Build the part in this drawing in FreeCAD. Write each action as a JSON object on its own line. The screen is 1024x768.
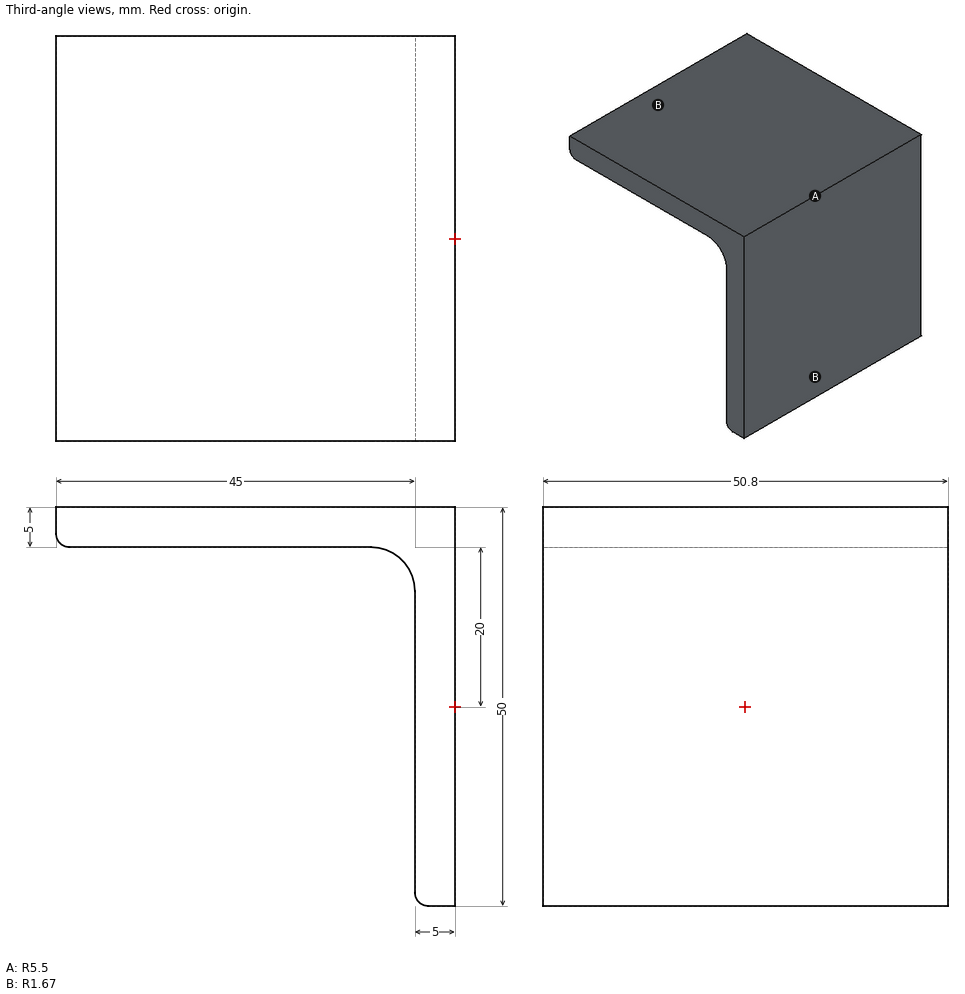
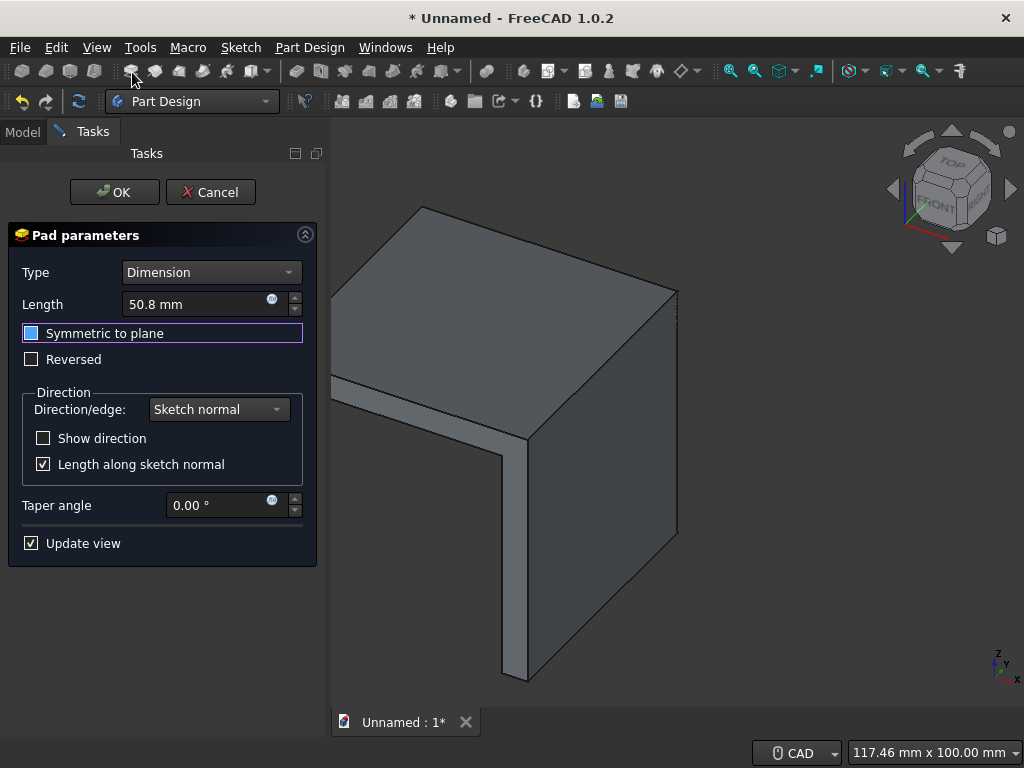
{"action": "left_click", "coordinate": [30, 333]}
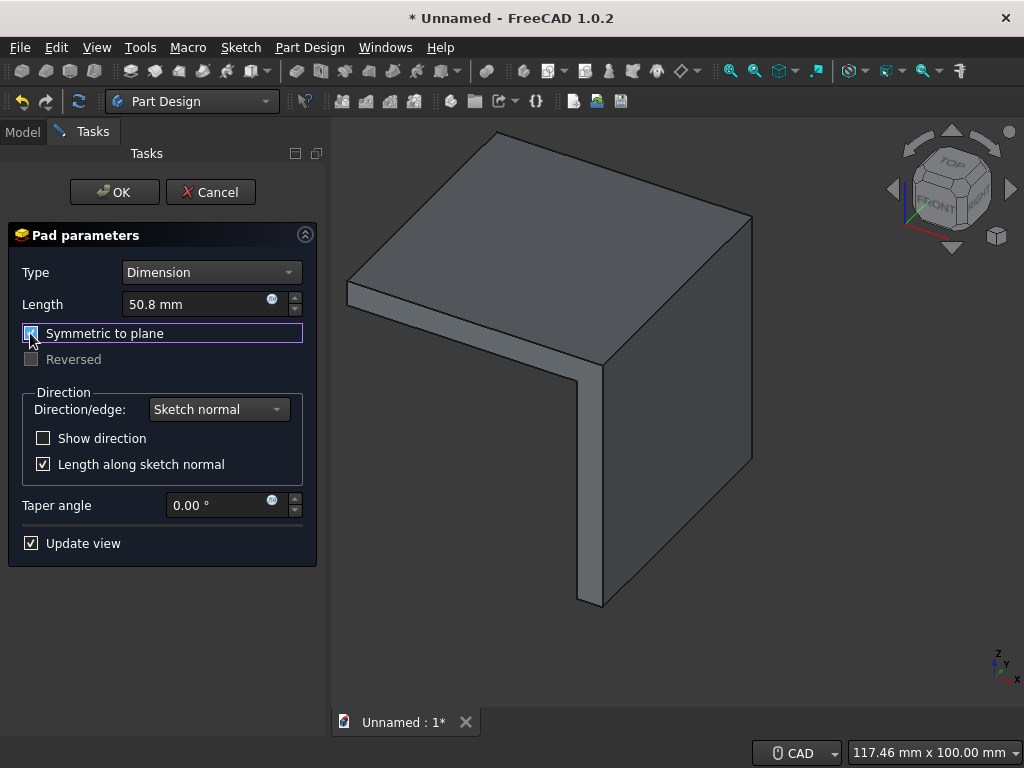
{"action": "left_click", "coordinate": [115, 192]}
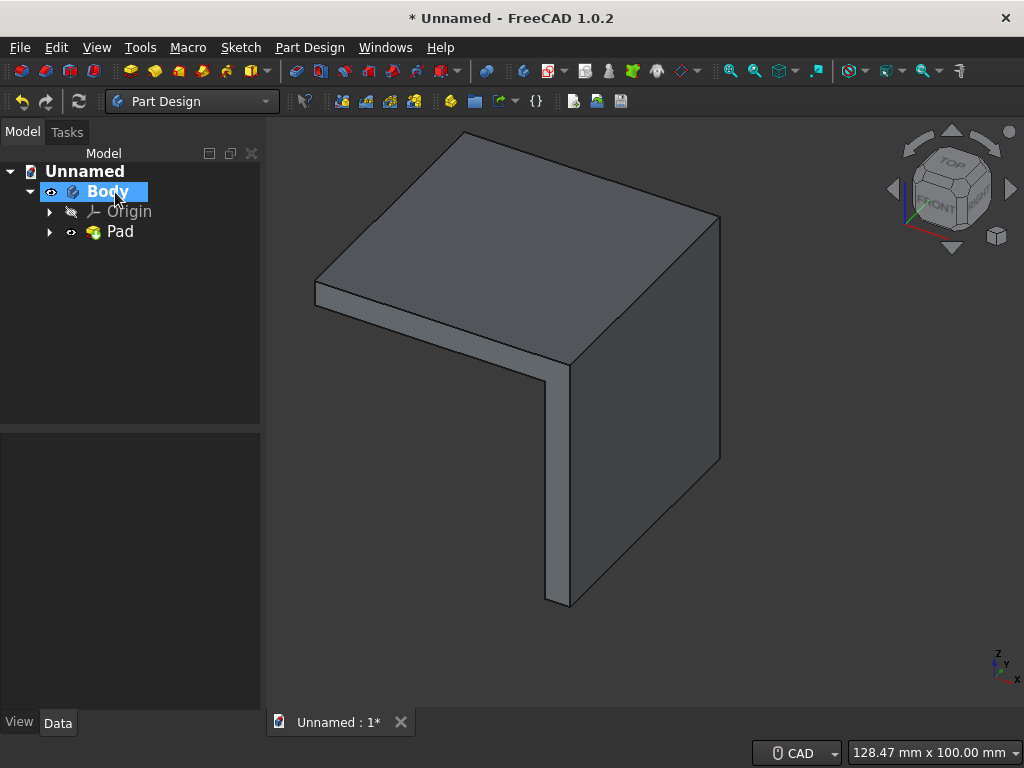
{"action": "key", "text": "0"}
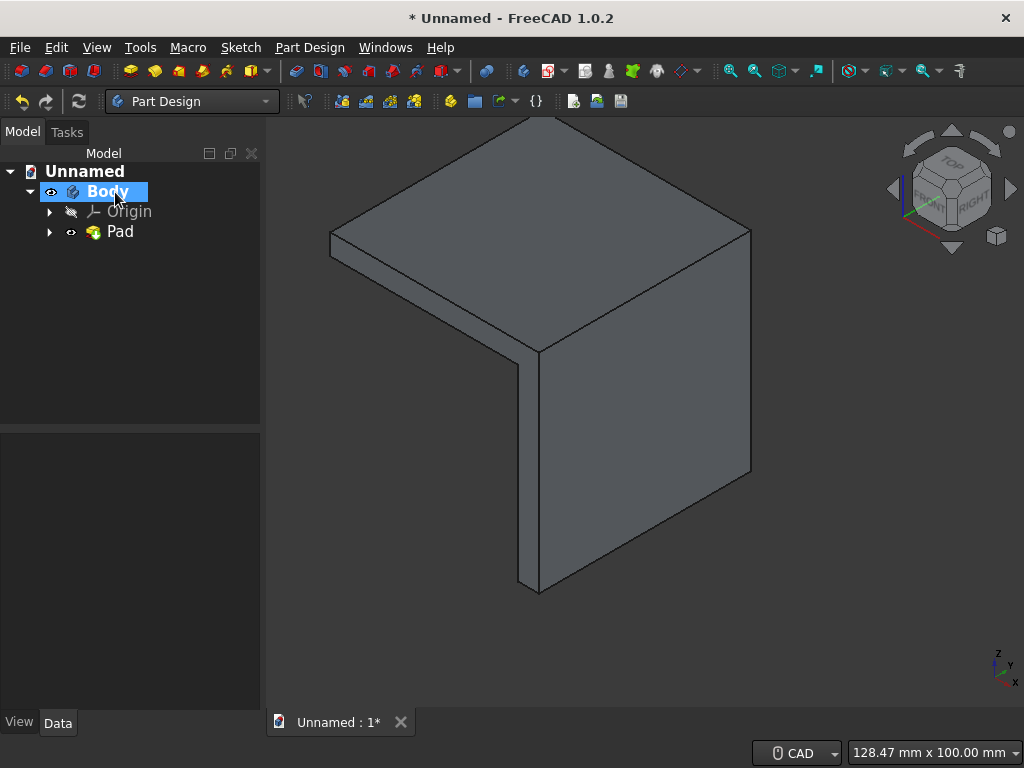
{"action": "left_click", "coordinate": [732, 72]}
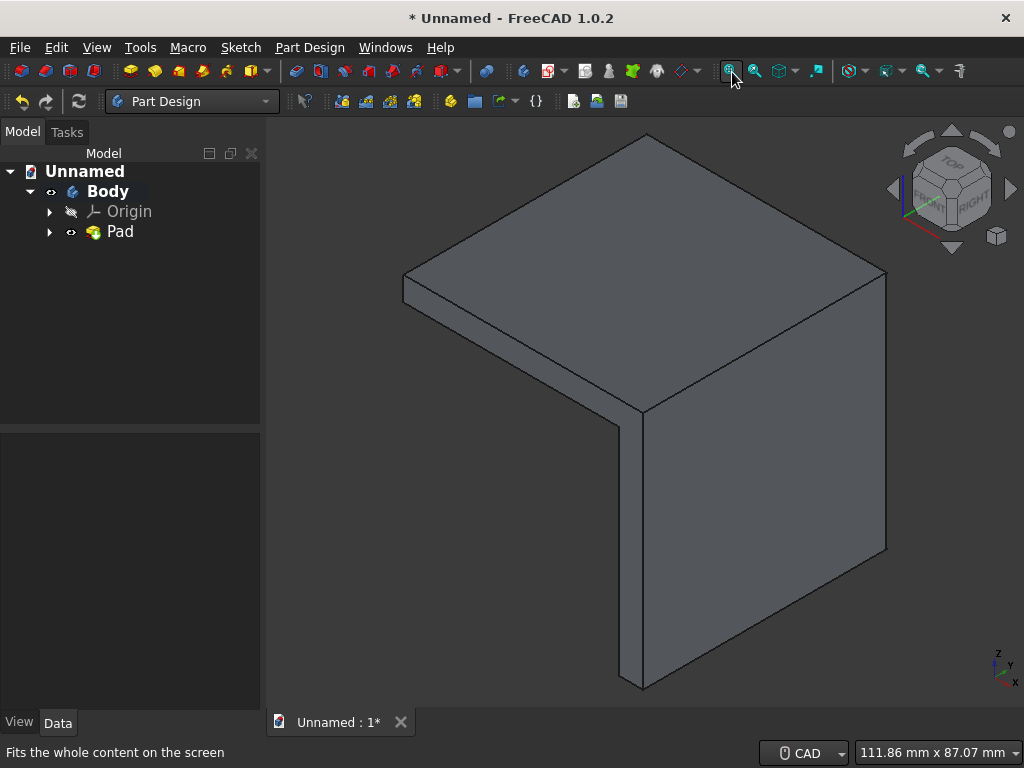
{"action": "key", "text": "2"}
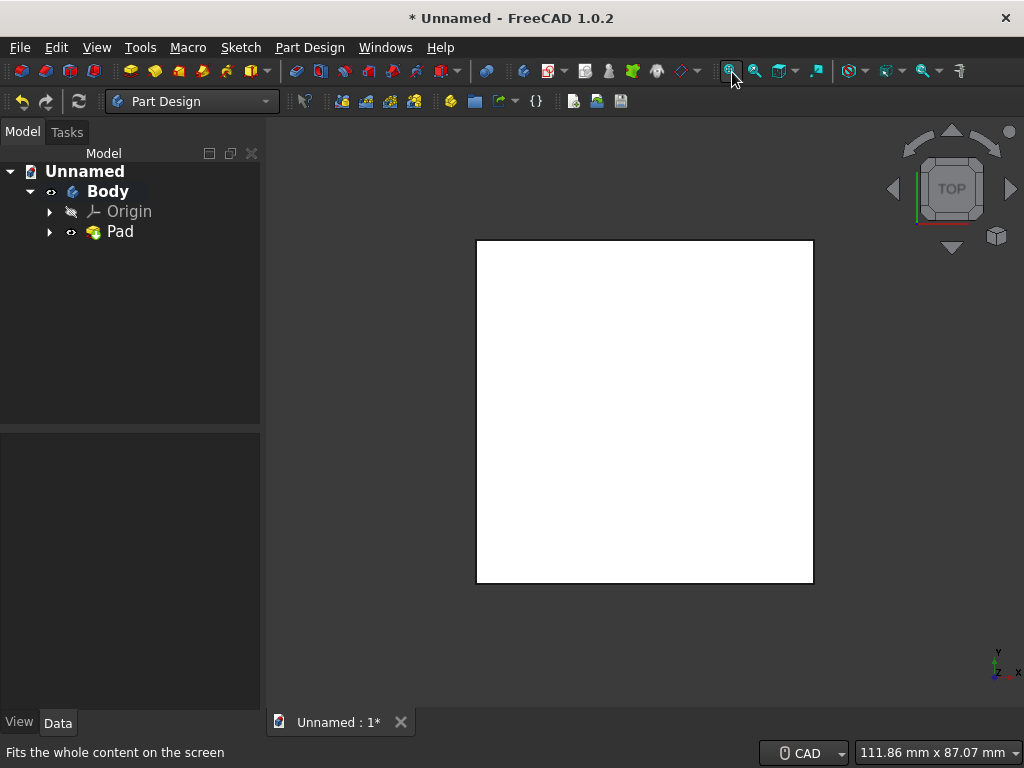
{"action": "key", "text": "1"}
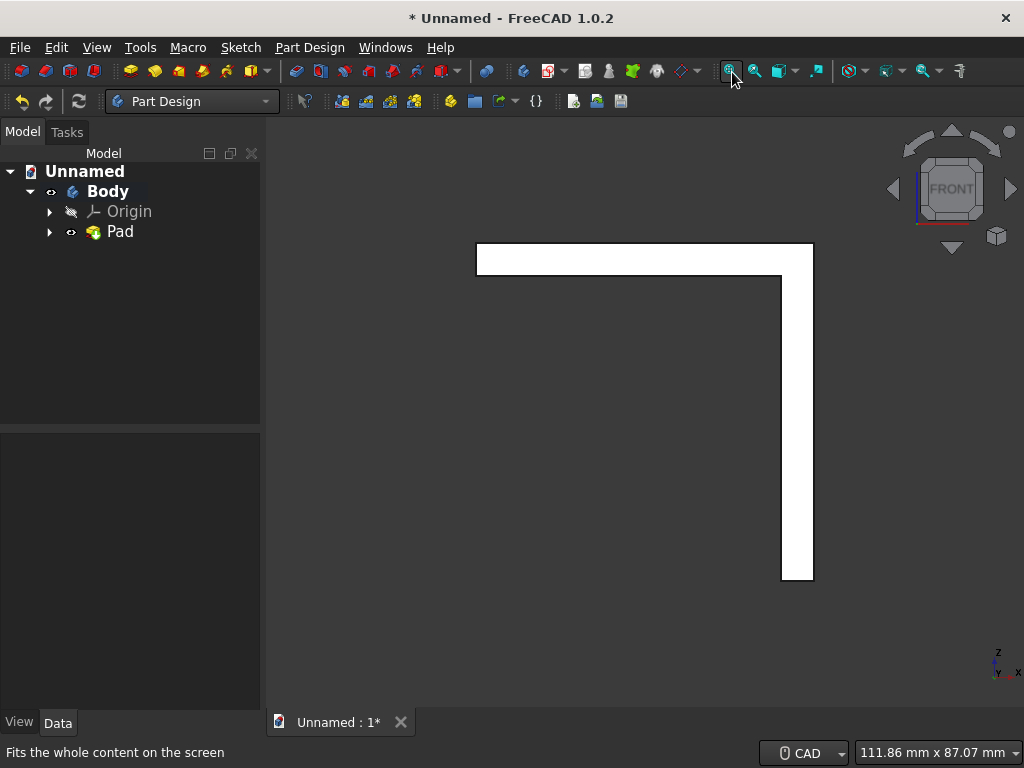
{"action": "key", "text": "3"}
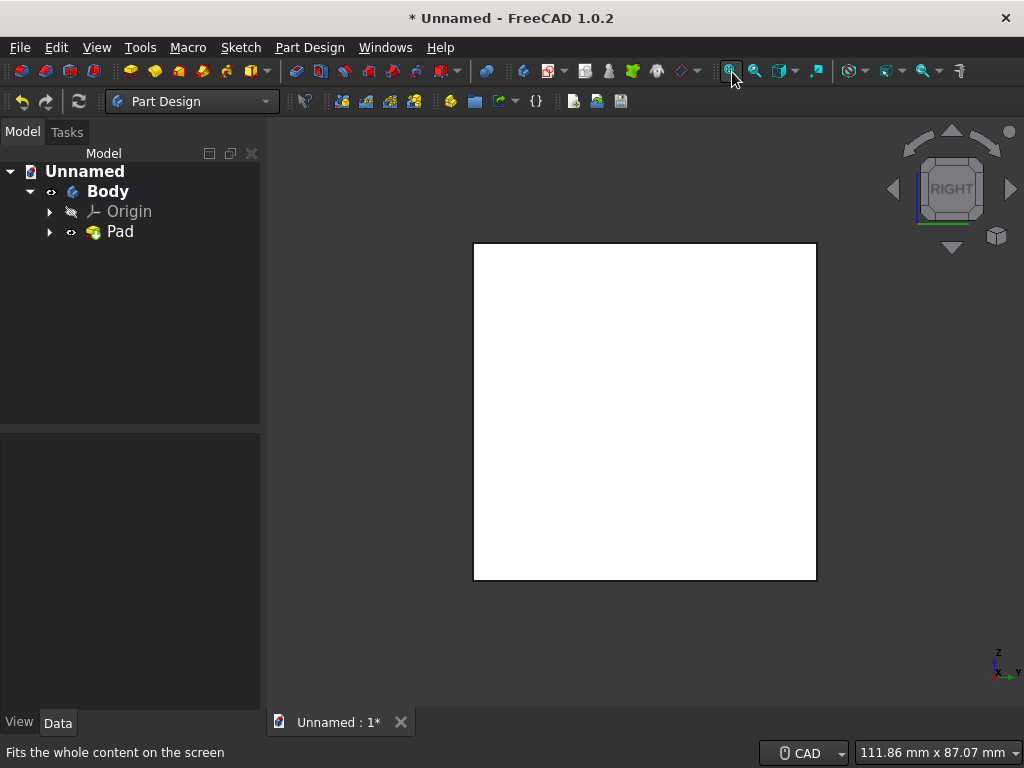
{"action": "key", "text": "5"}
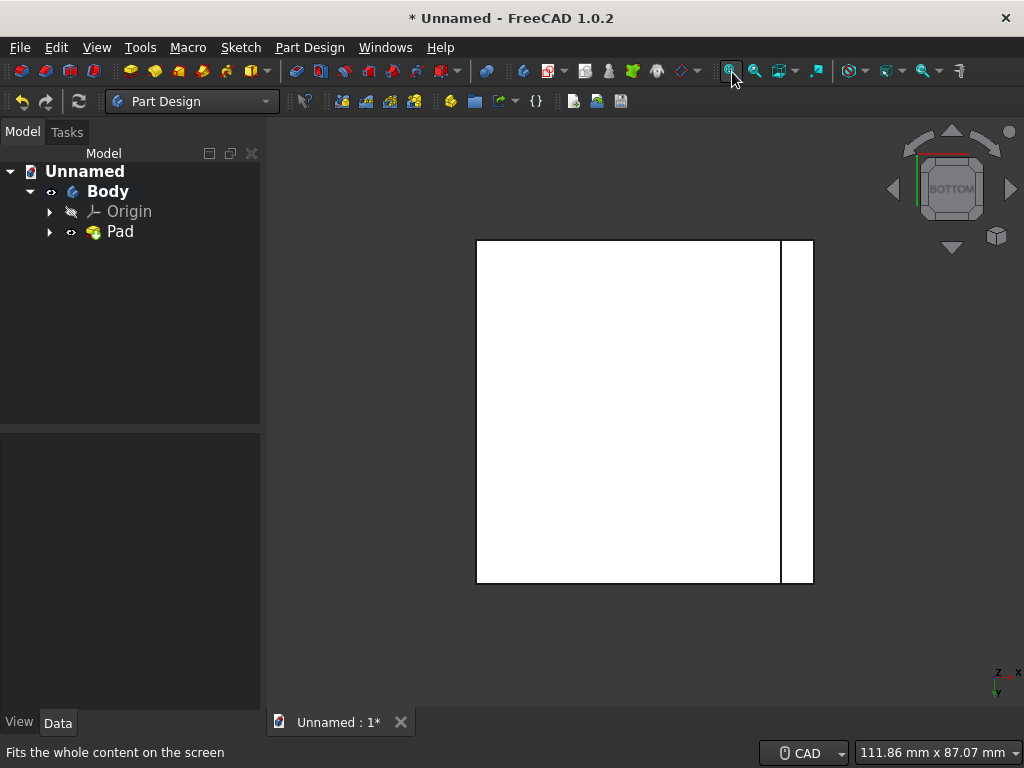
{"action": "key", "text": "4"}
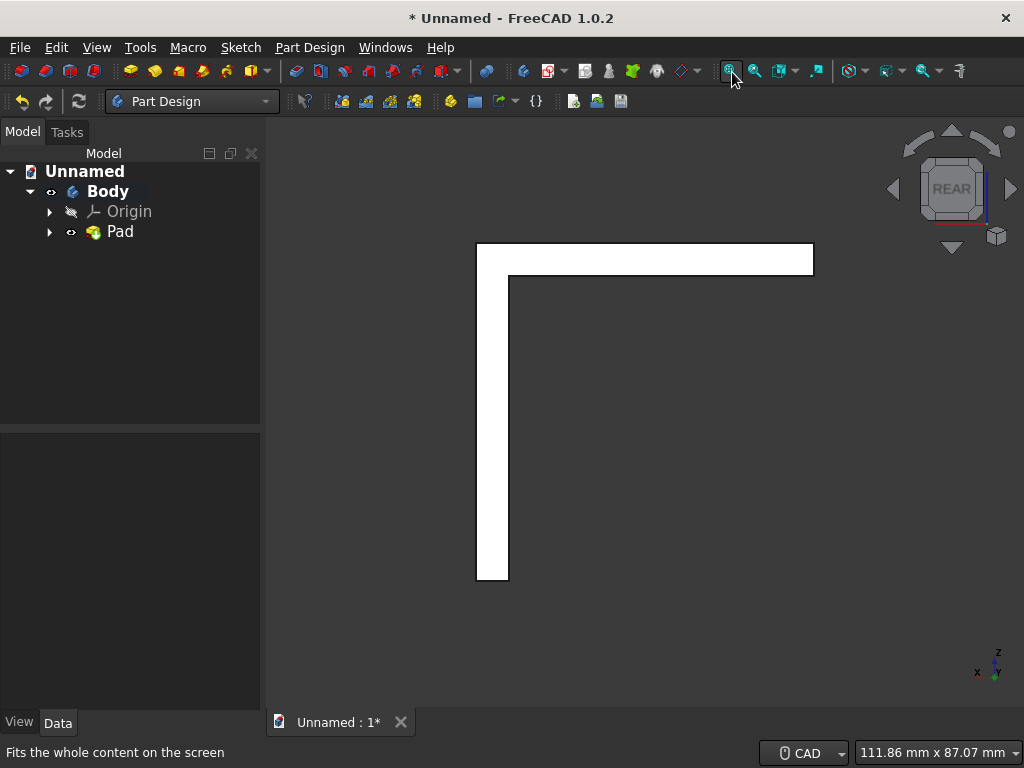
{"action": "key", "text": "6"}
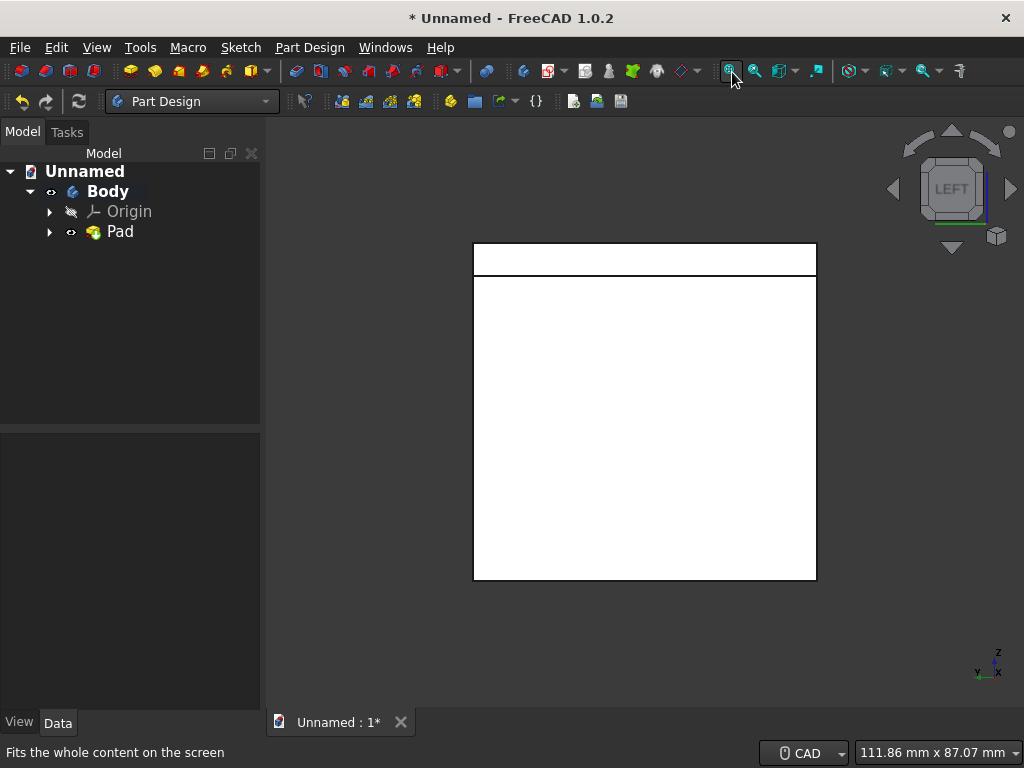
{"action": "key", "text": "v 3"}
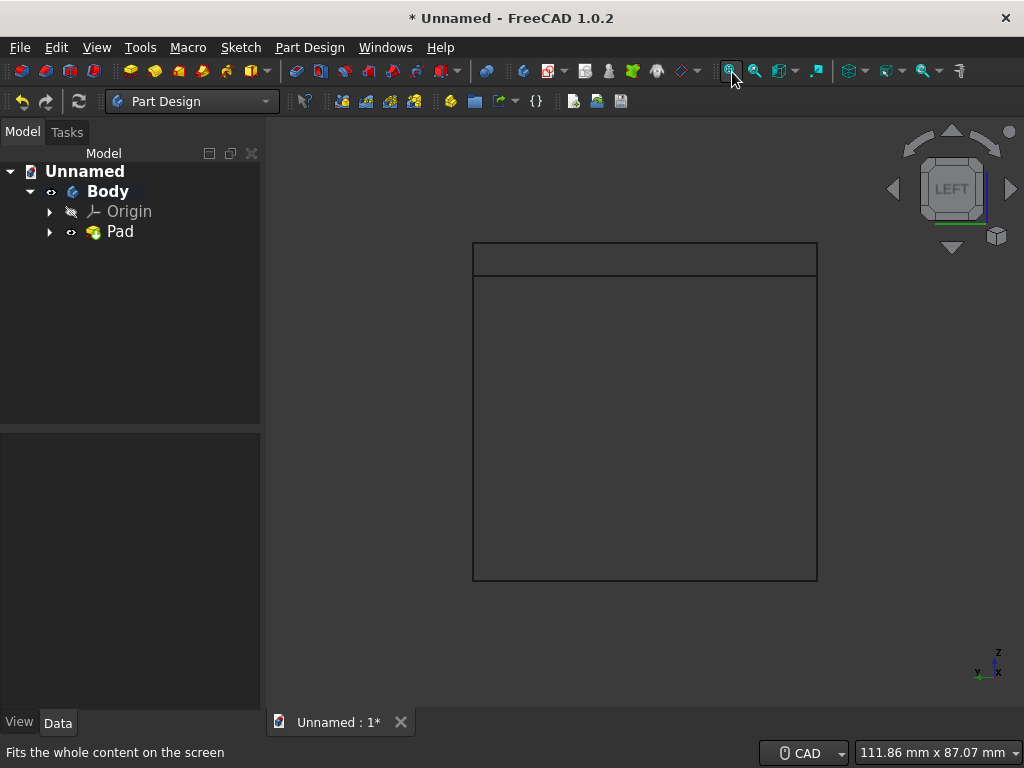
{"action": "key", "text": "0"}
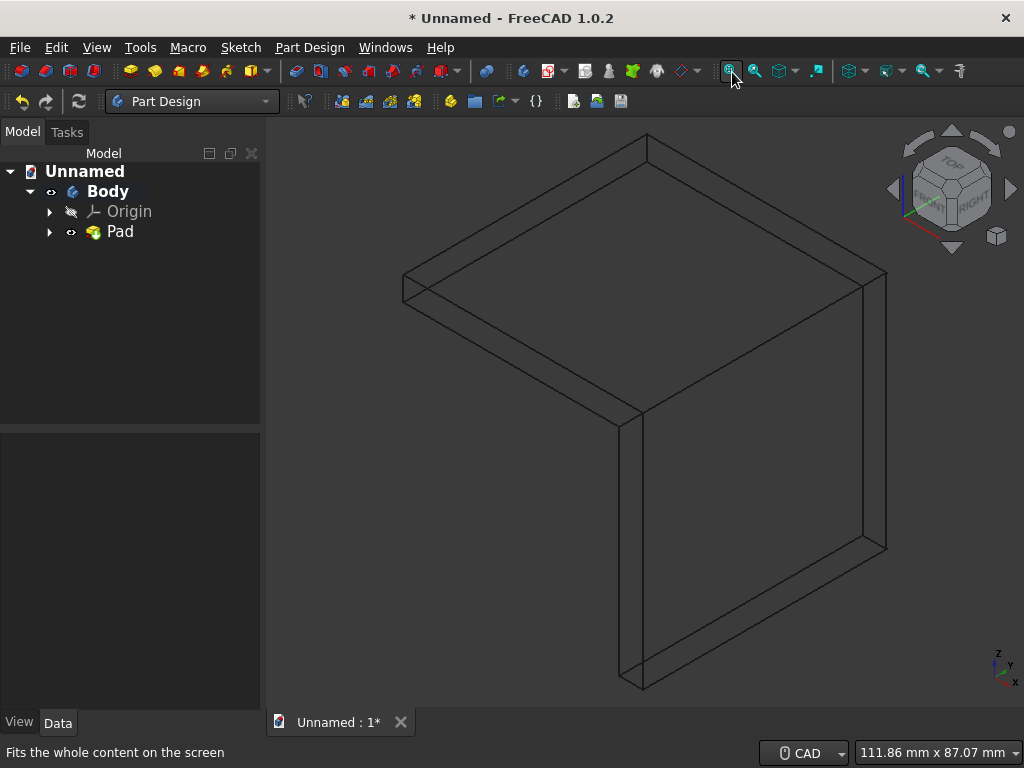
{"action": "scroll", "coordinate": [741, 356], "scroll_direction": "up", "scroll_amount": 6}